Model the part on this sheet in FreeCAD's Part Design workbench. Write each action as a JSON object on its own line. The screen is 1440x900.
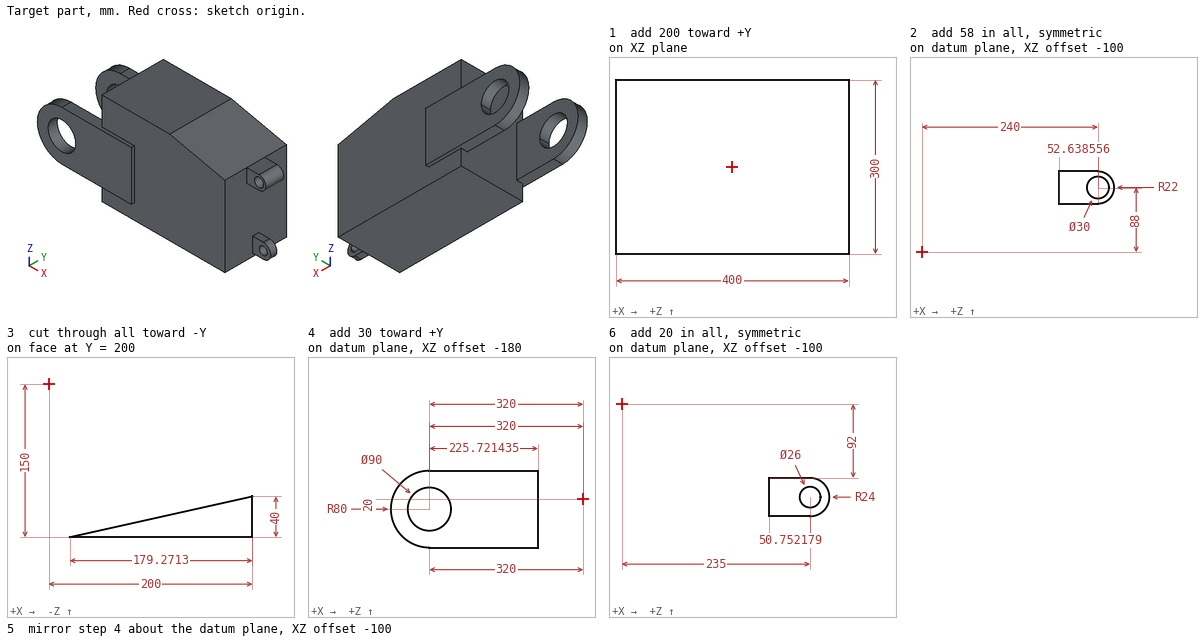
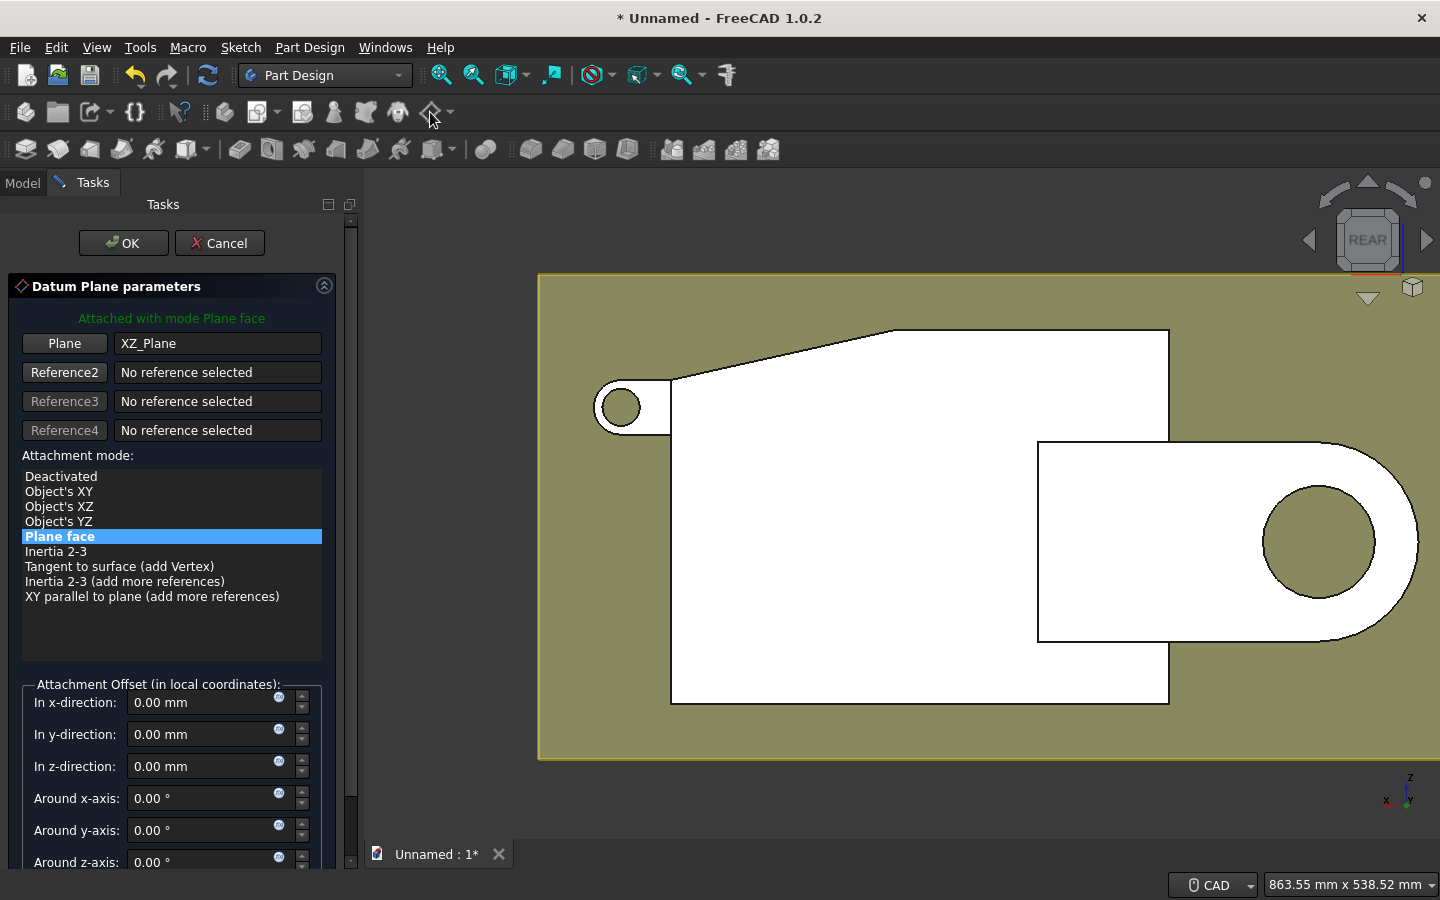
{"action": "triple_click", "coordinate": [210, 766]}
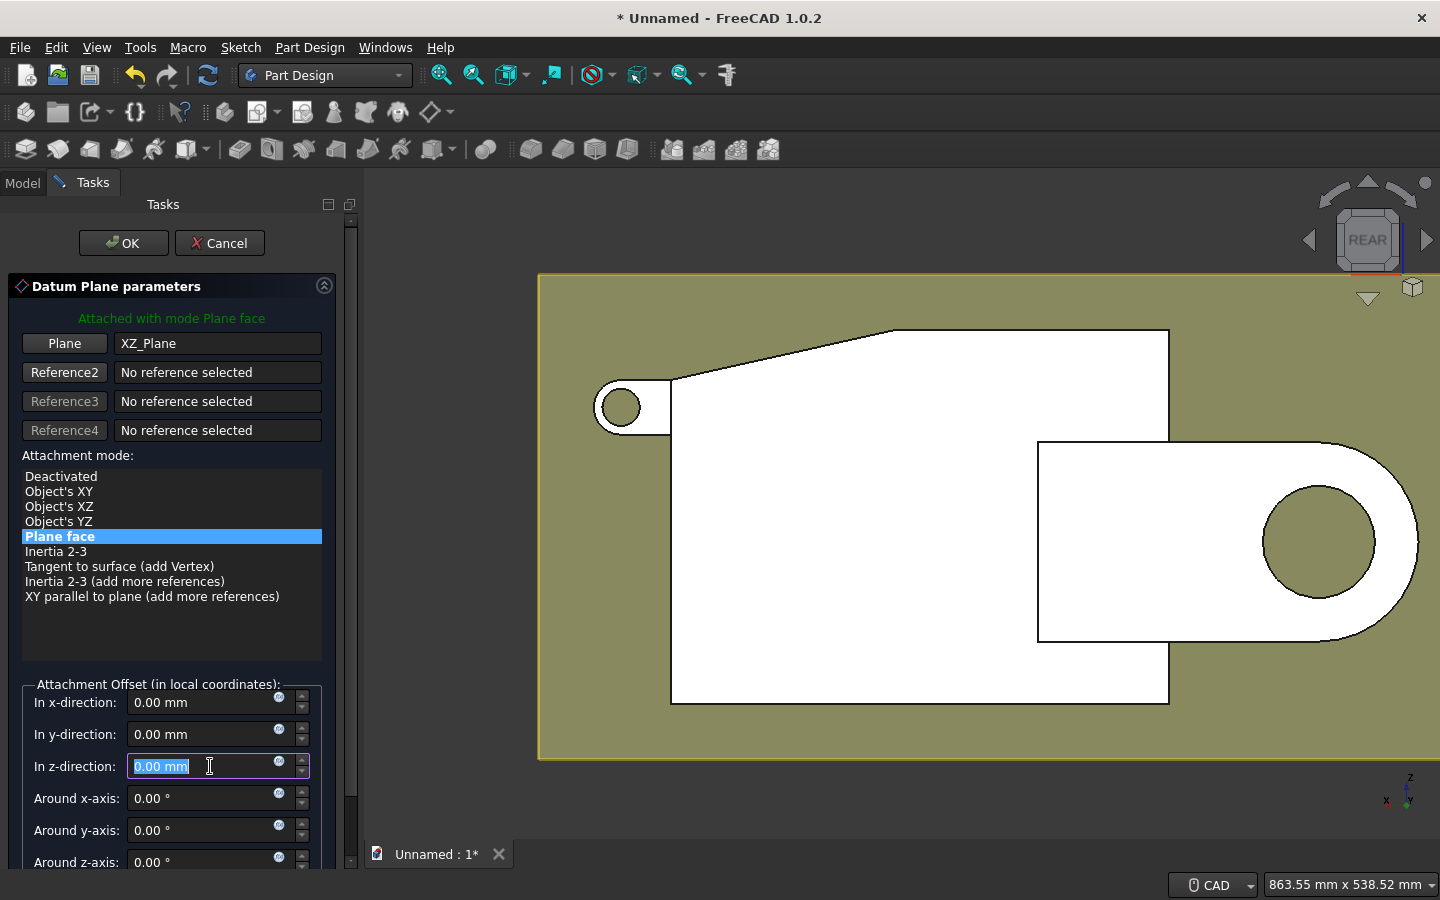
{"action": "type", "text": "-100"}
{"action": "key", "text": "Tab"}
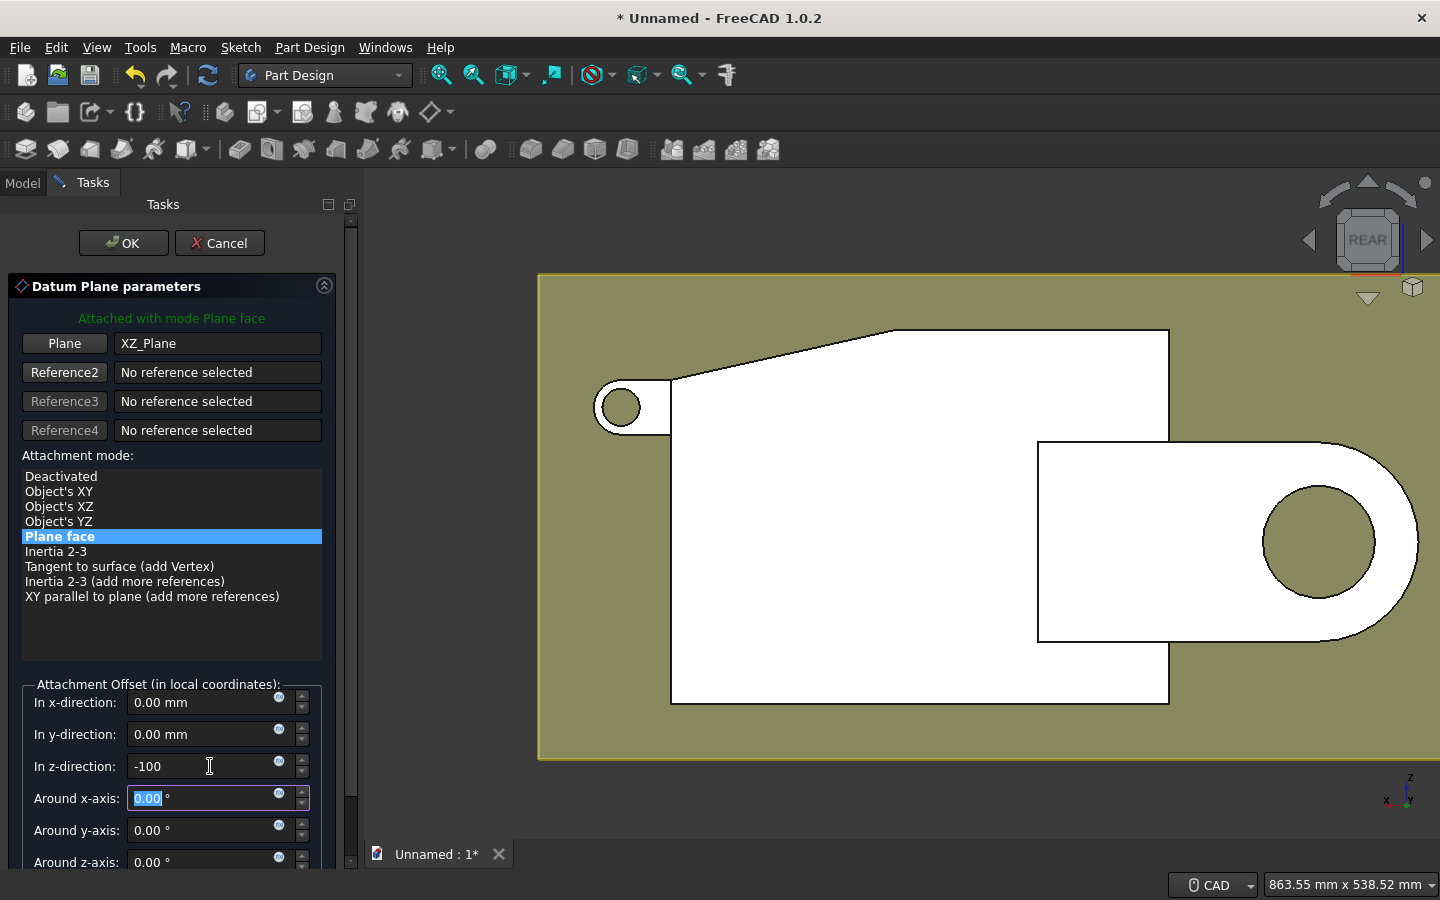
{"action": "left_click", "coordinate": [124, 243]}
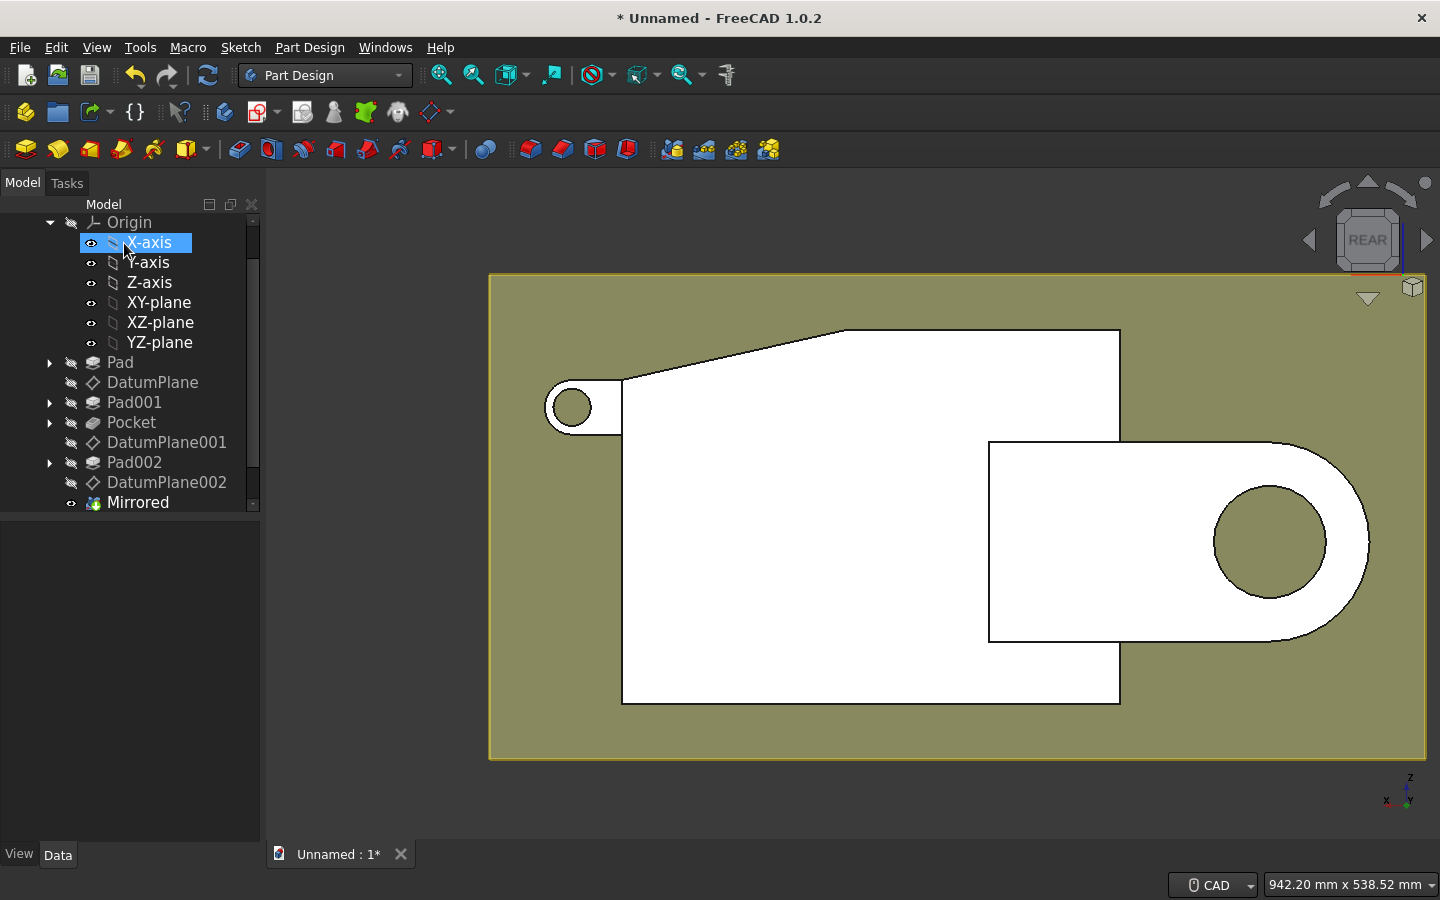
{"action": "scroll", "coordinate": [140, 358], "scroll_direction": "down", "scroll_amount": 3}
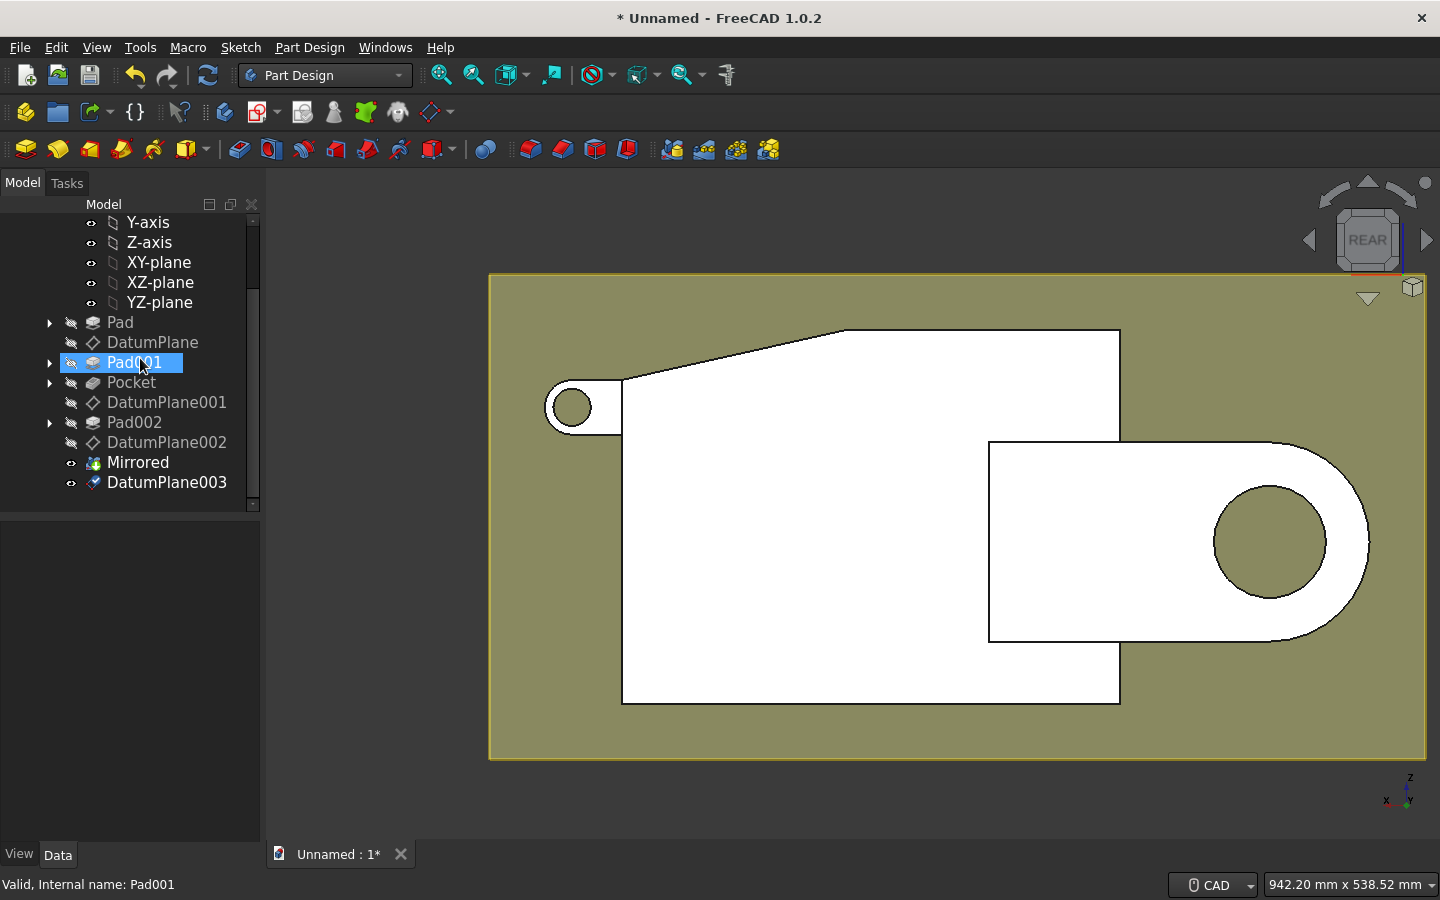
{"action": "left_click", "coordinate": [116, 483]}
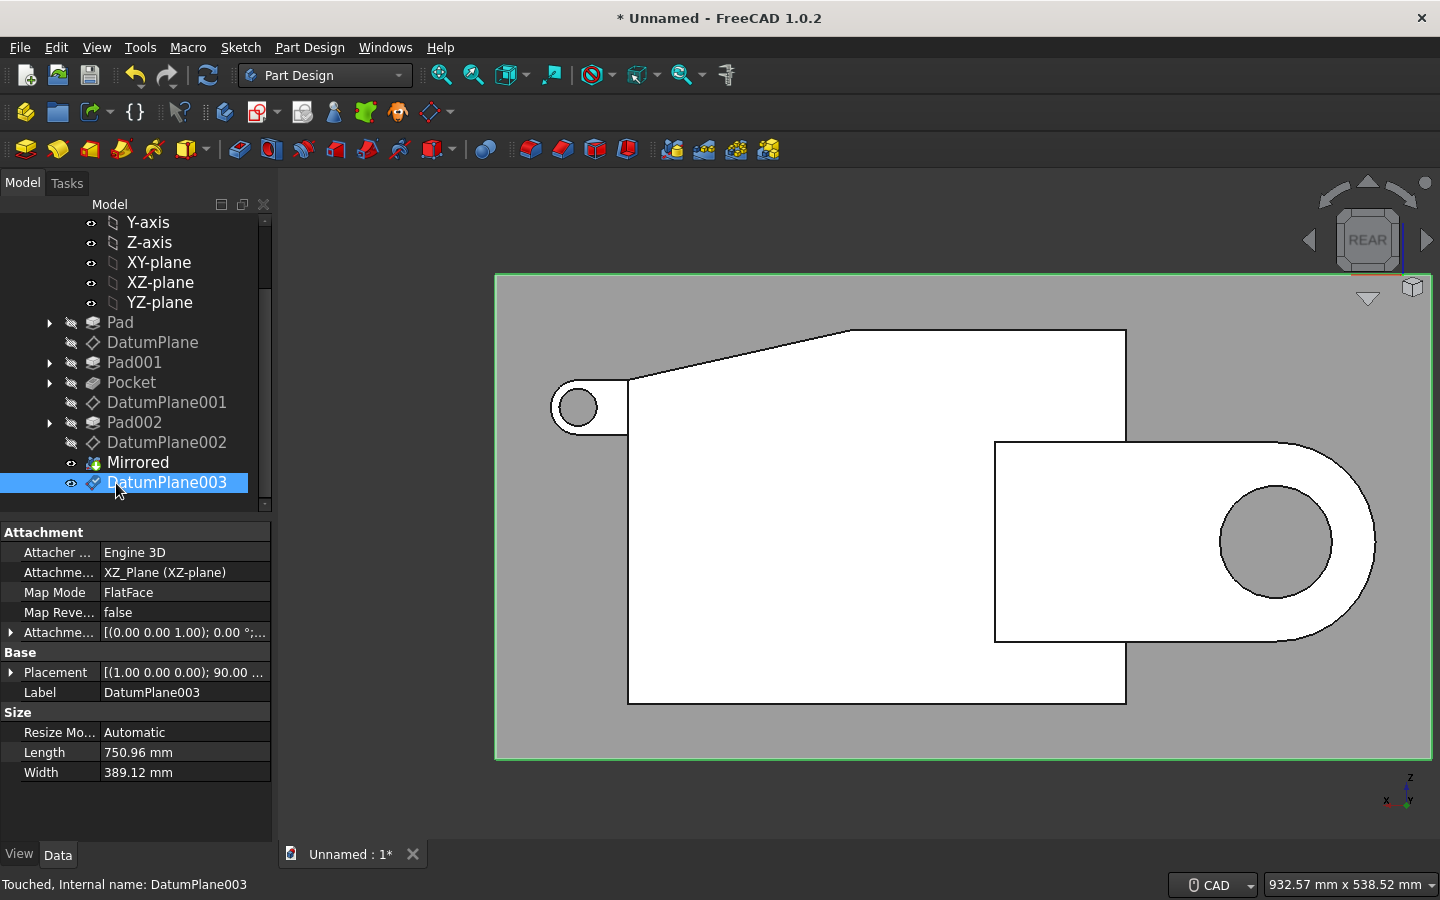
{"action": "left_click", "coordinate": [258, 112]}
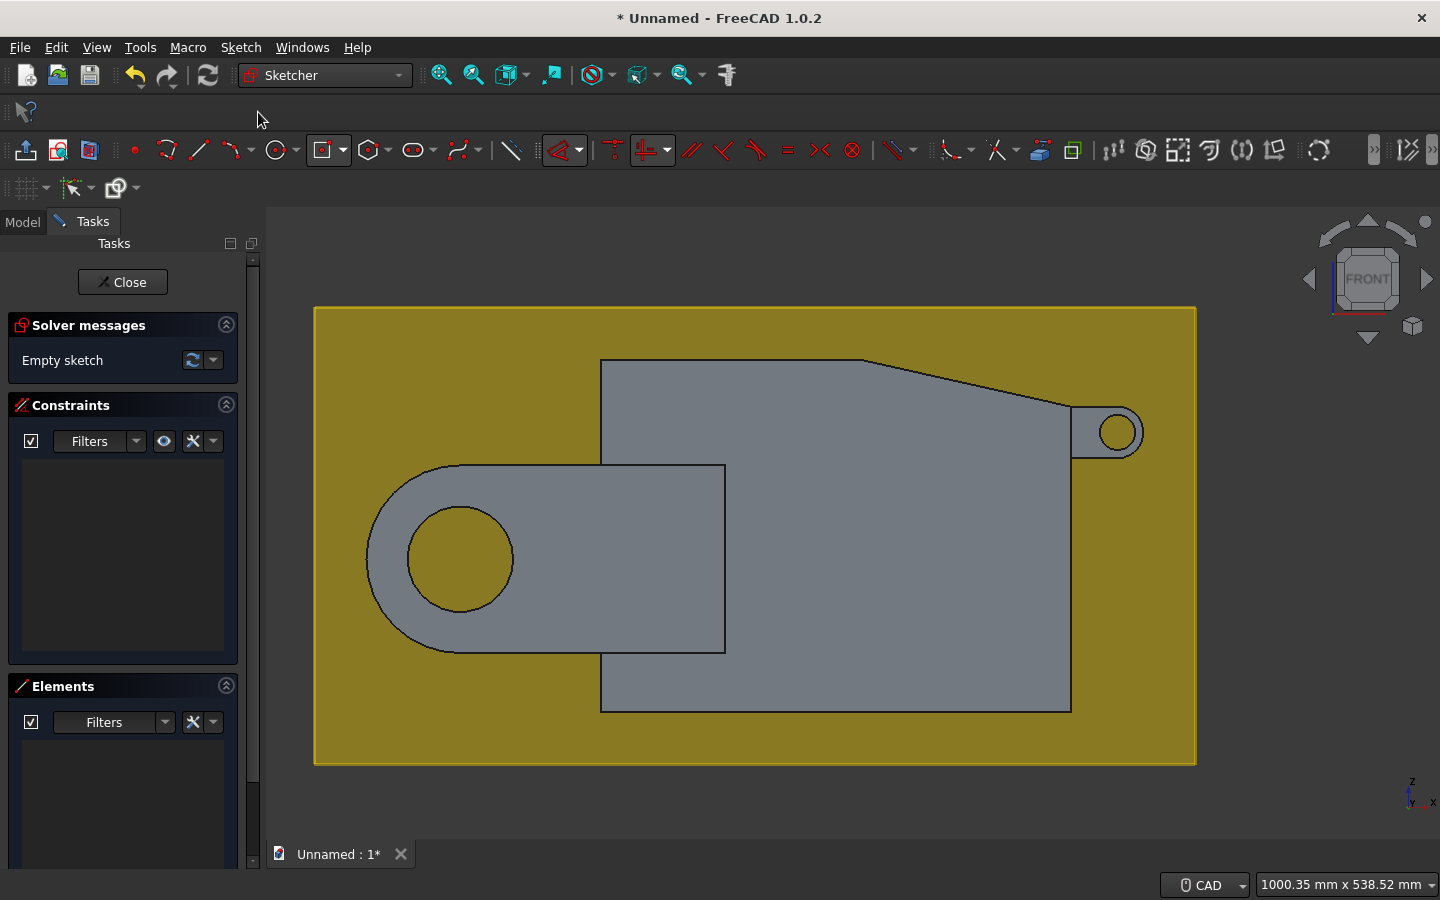
{"action": "left_click", "coordinate": [90, 150]}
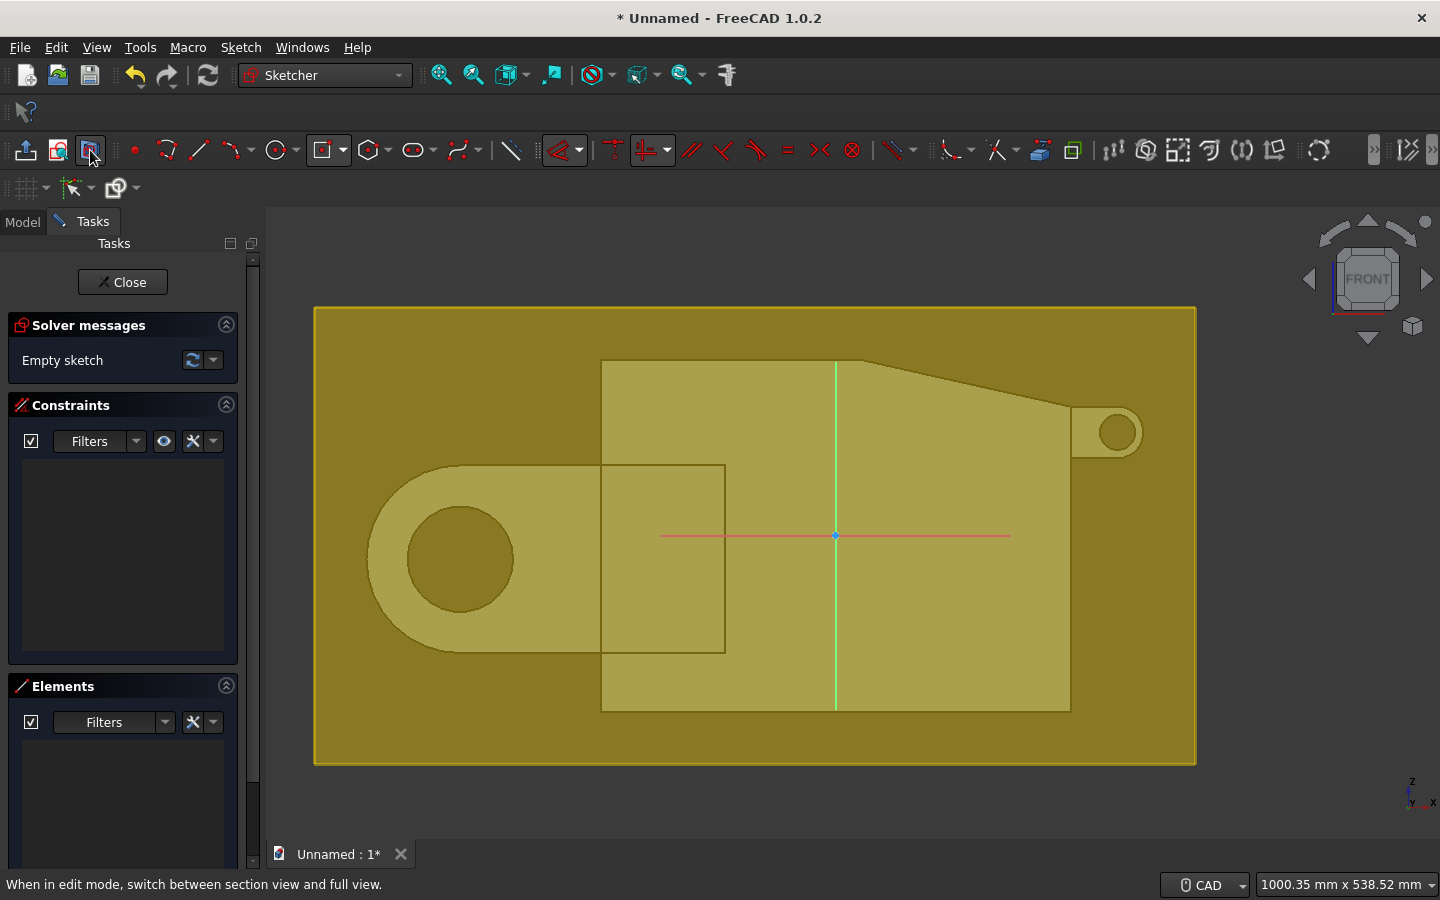
{"action": "scroll", "coordinate": [1145, 695], "scroll_direction": "up", "scroll_amount": 10}